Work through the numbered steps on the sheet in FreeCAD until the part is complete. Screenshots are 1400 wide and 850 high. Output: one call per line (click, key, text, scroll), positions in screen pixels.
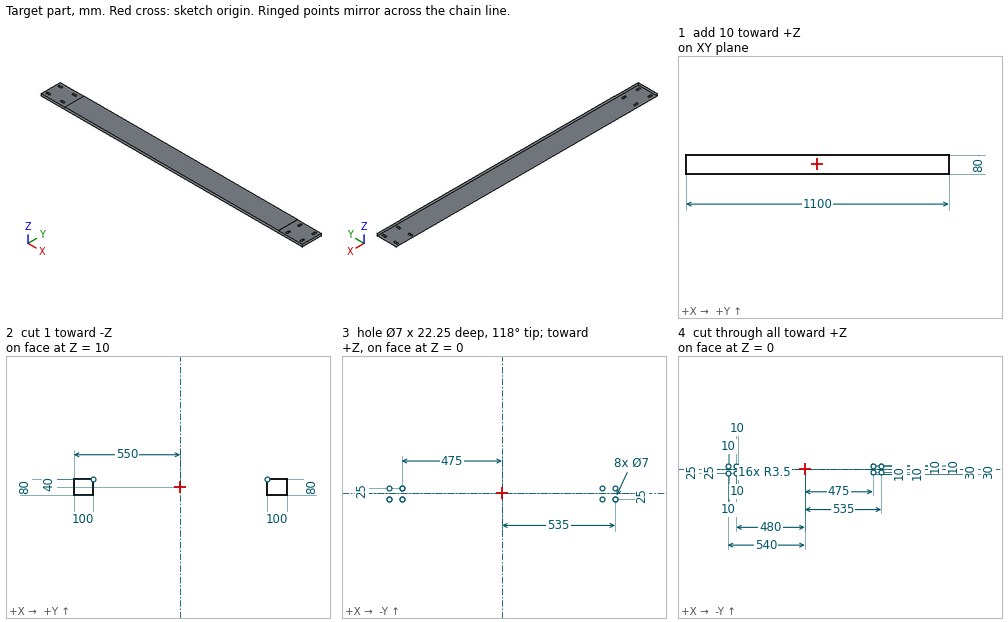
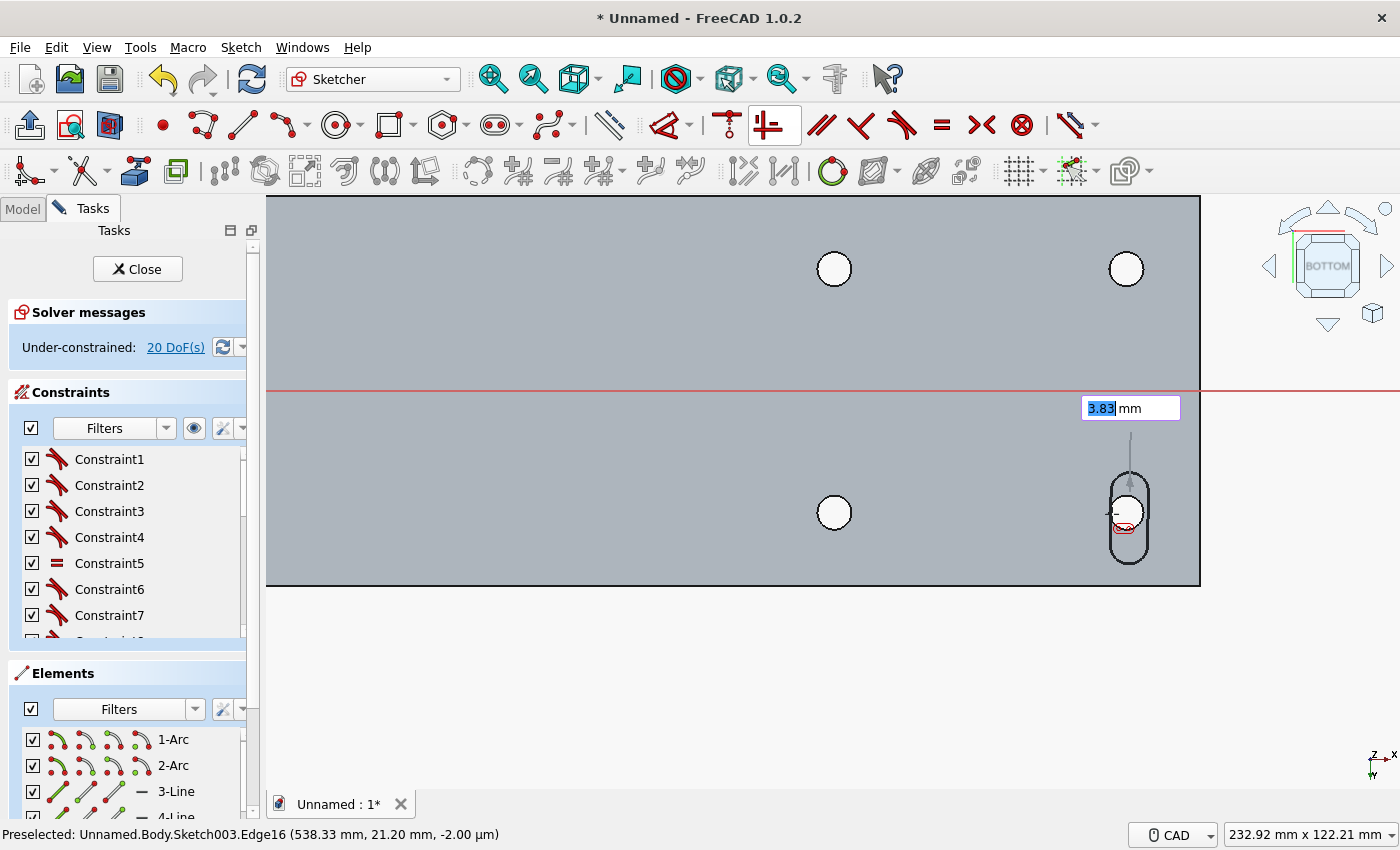
click(1109, 513)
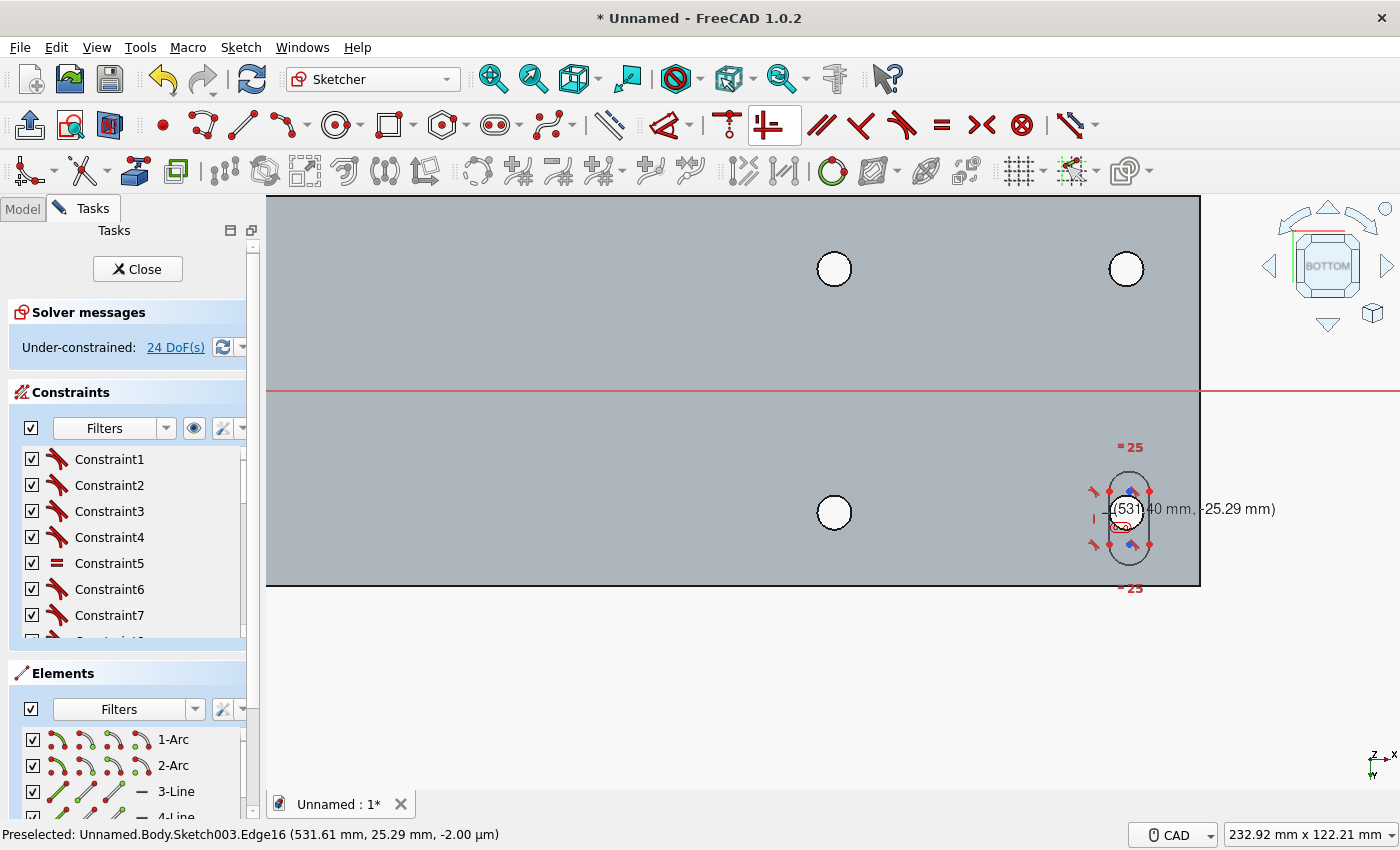
scroll(834, 537, up, 2)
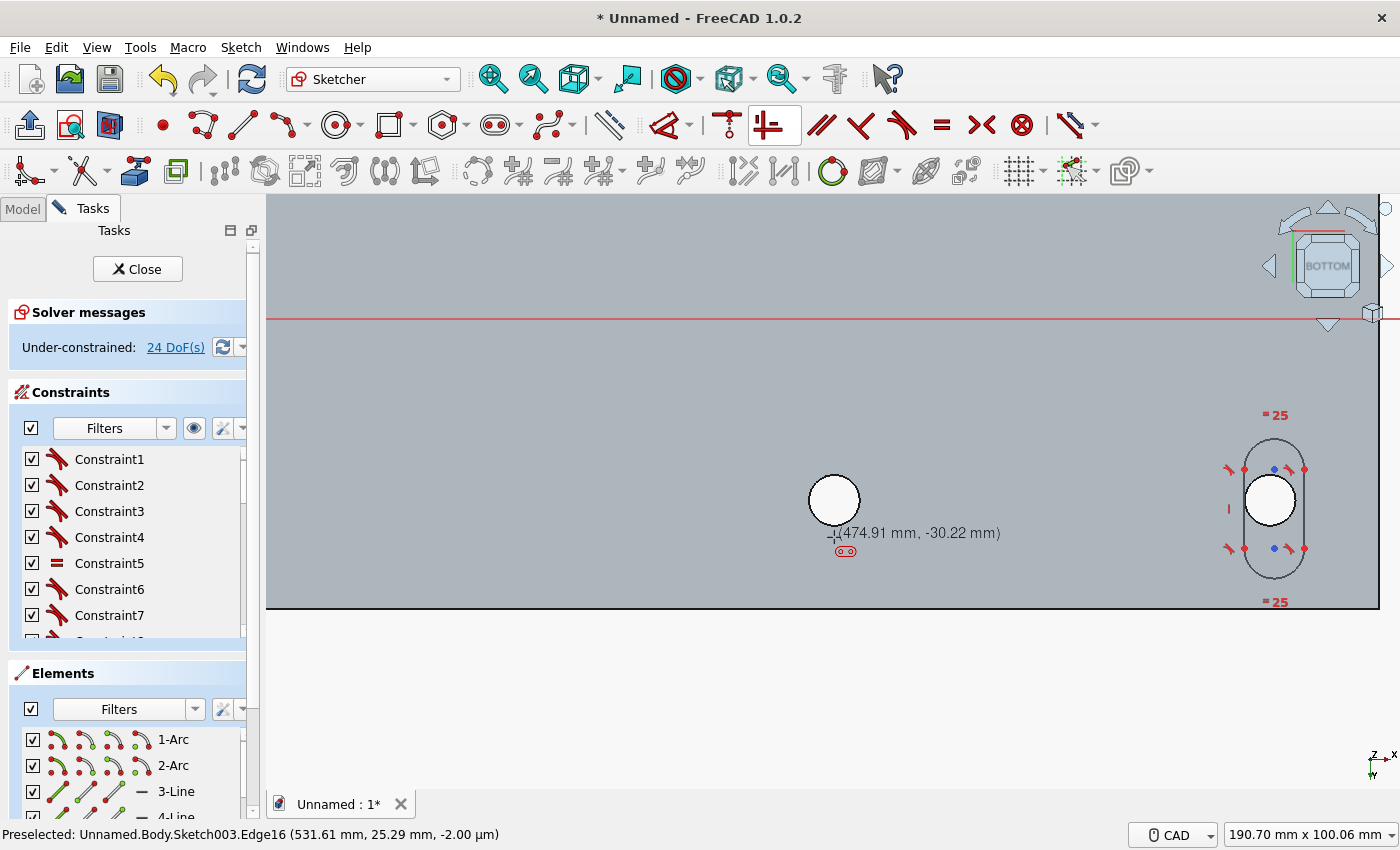
scroll(1104, 509, down, 12)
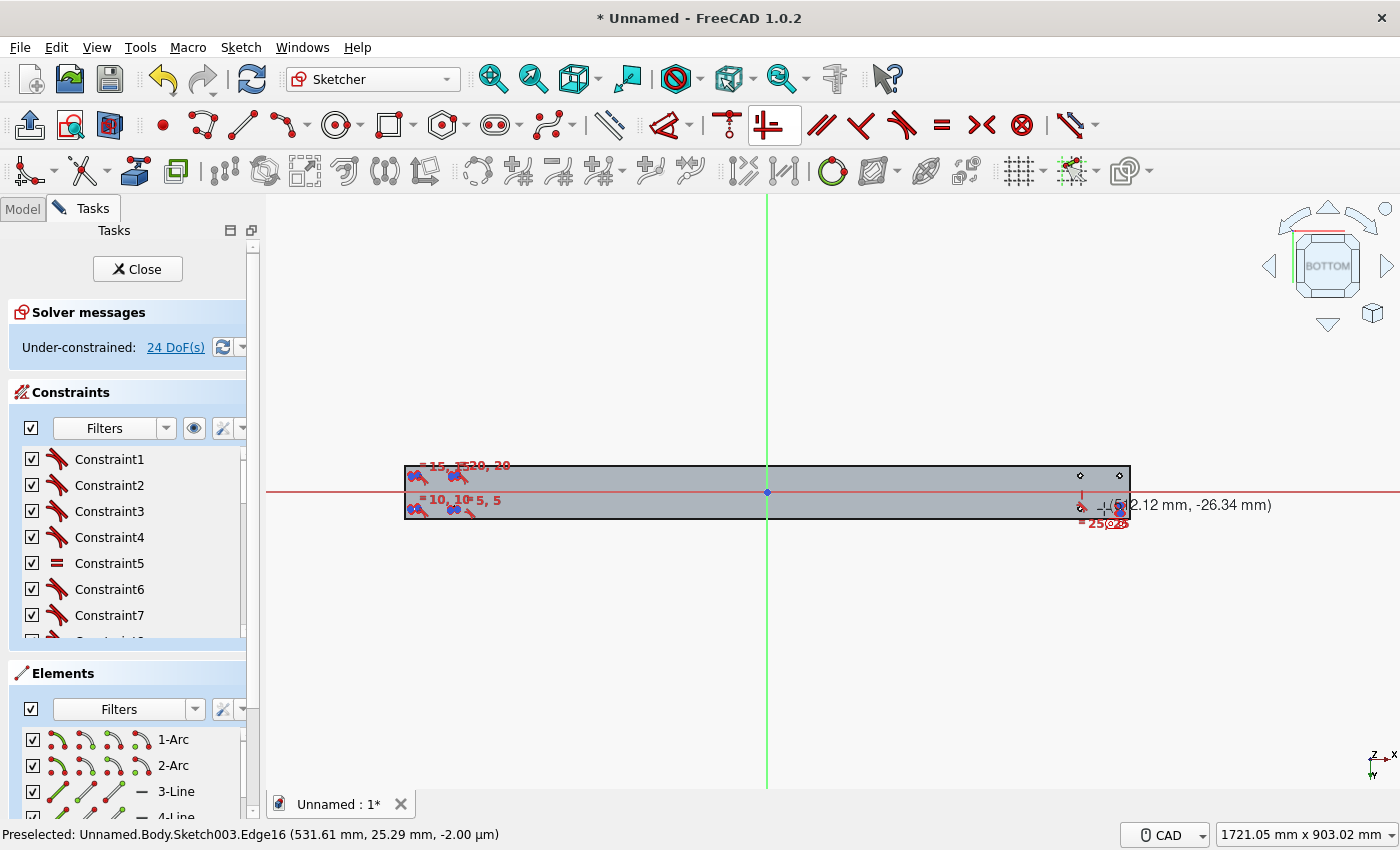
click(1080, 512)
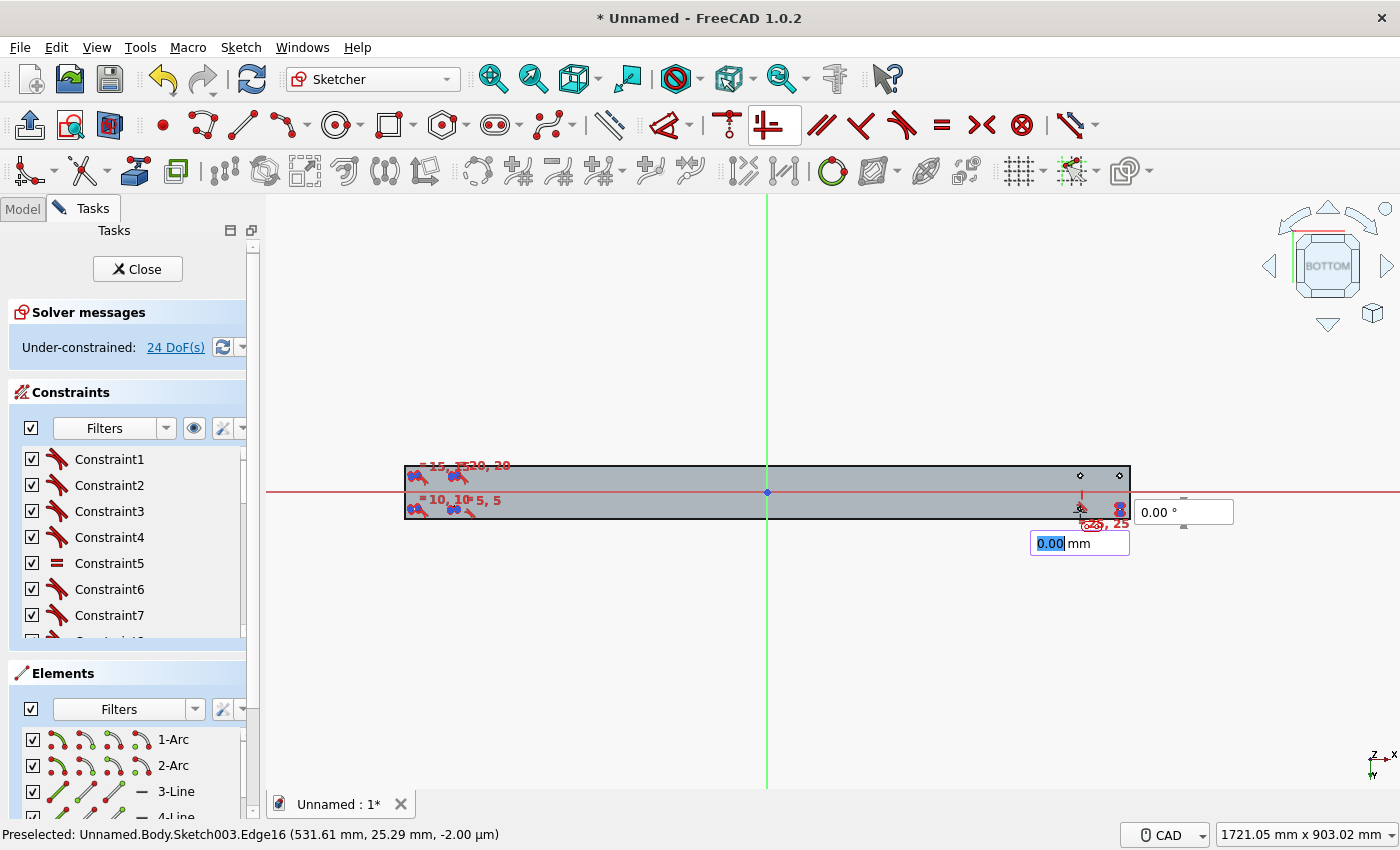
scroll(1080, 505, up, 5)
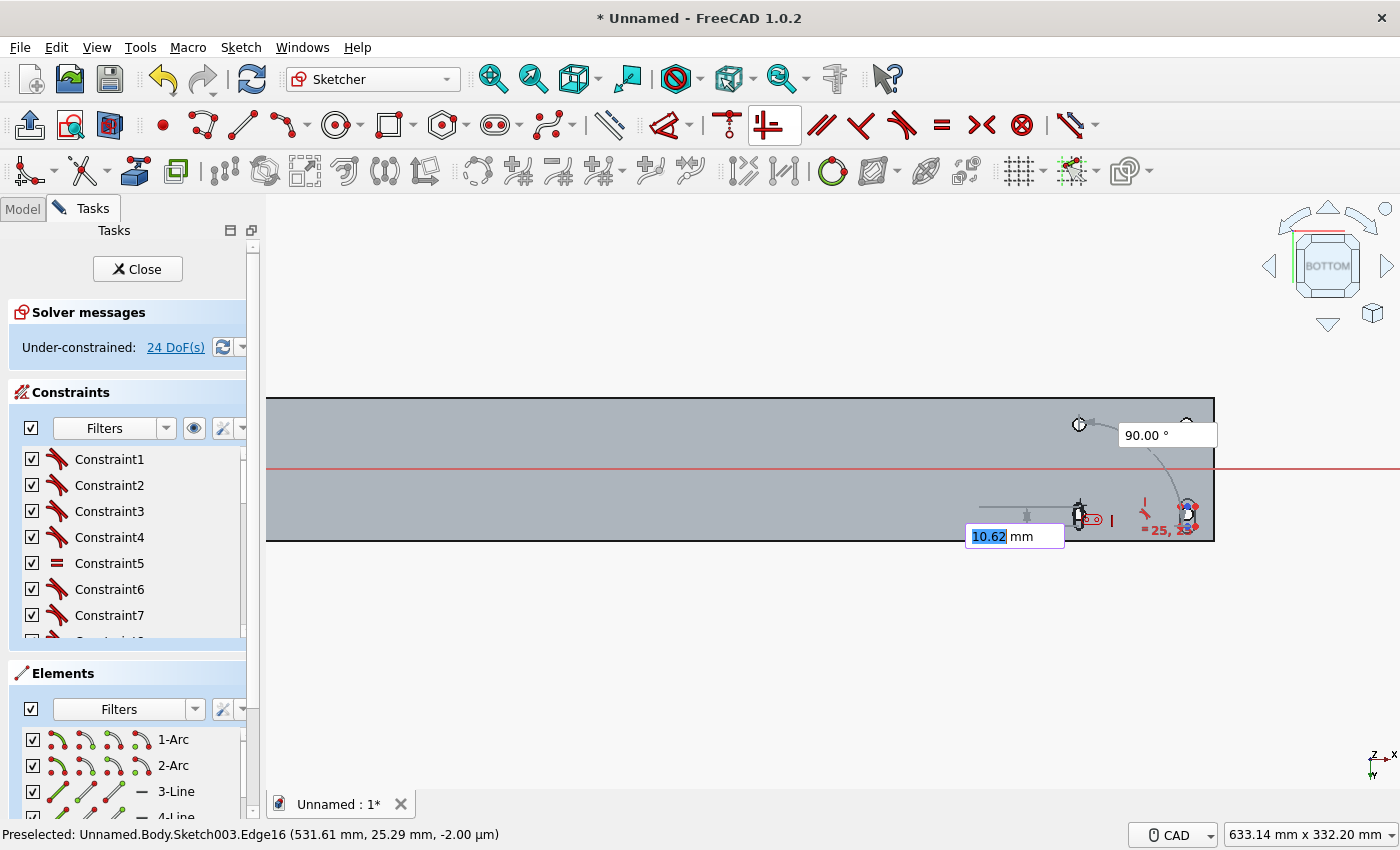
click(1079, 505)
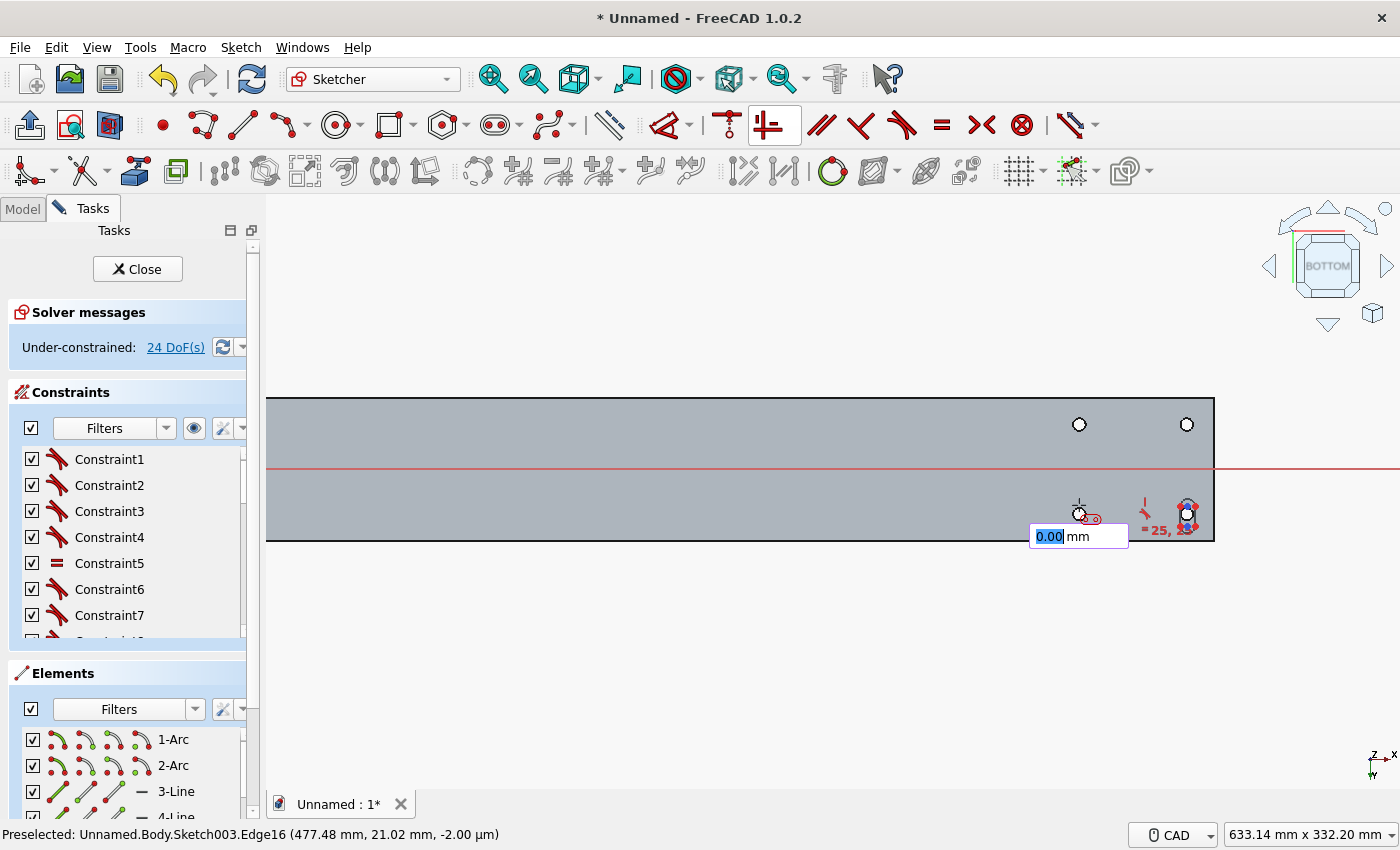
scroll(1073, 514, up, 5)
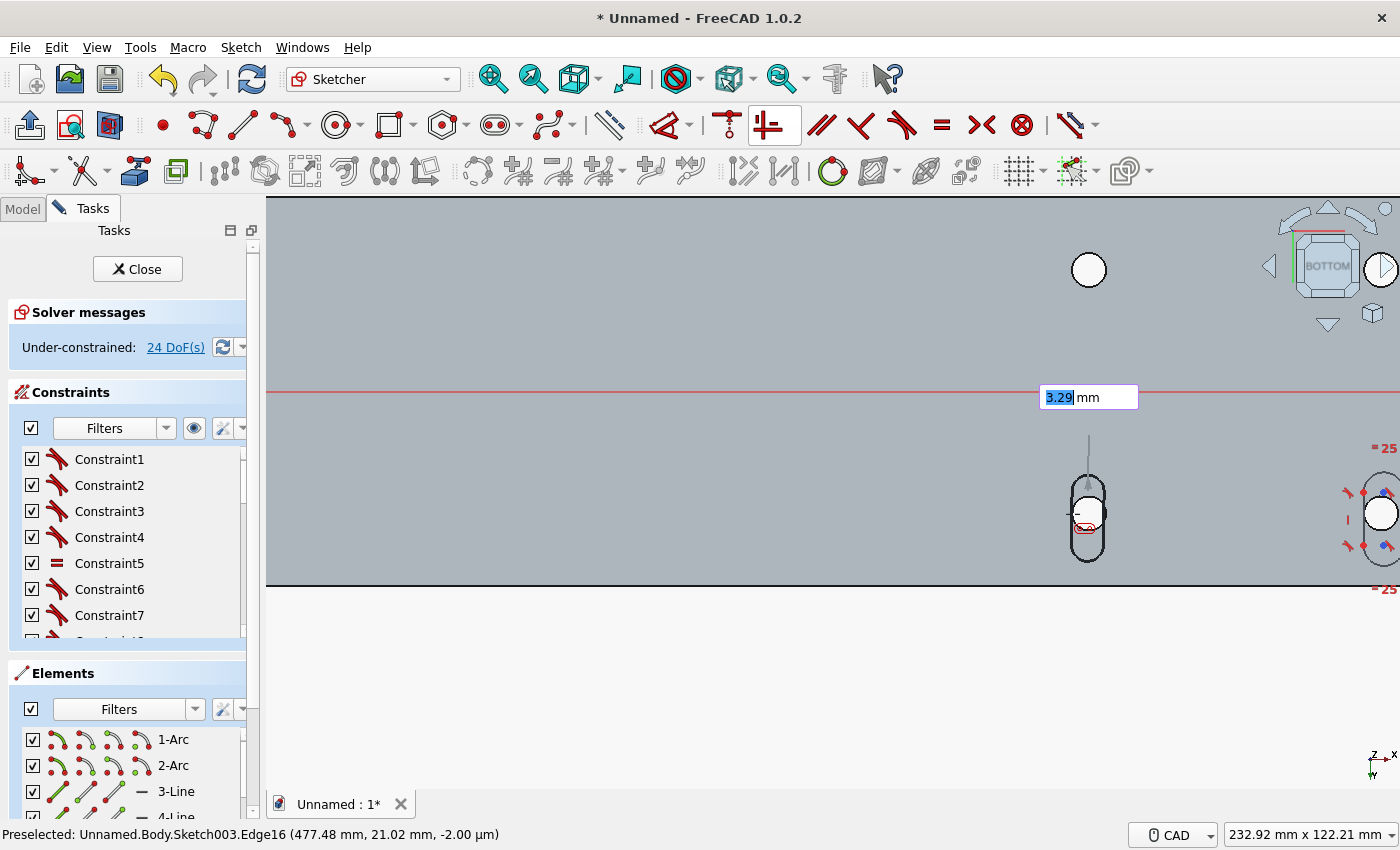
click(1072, 513)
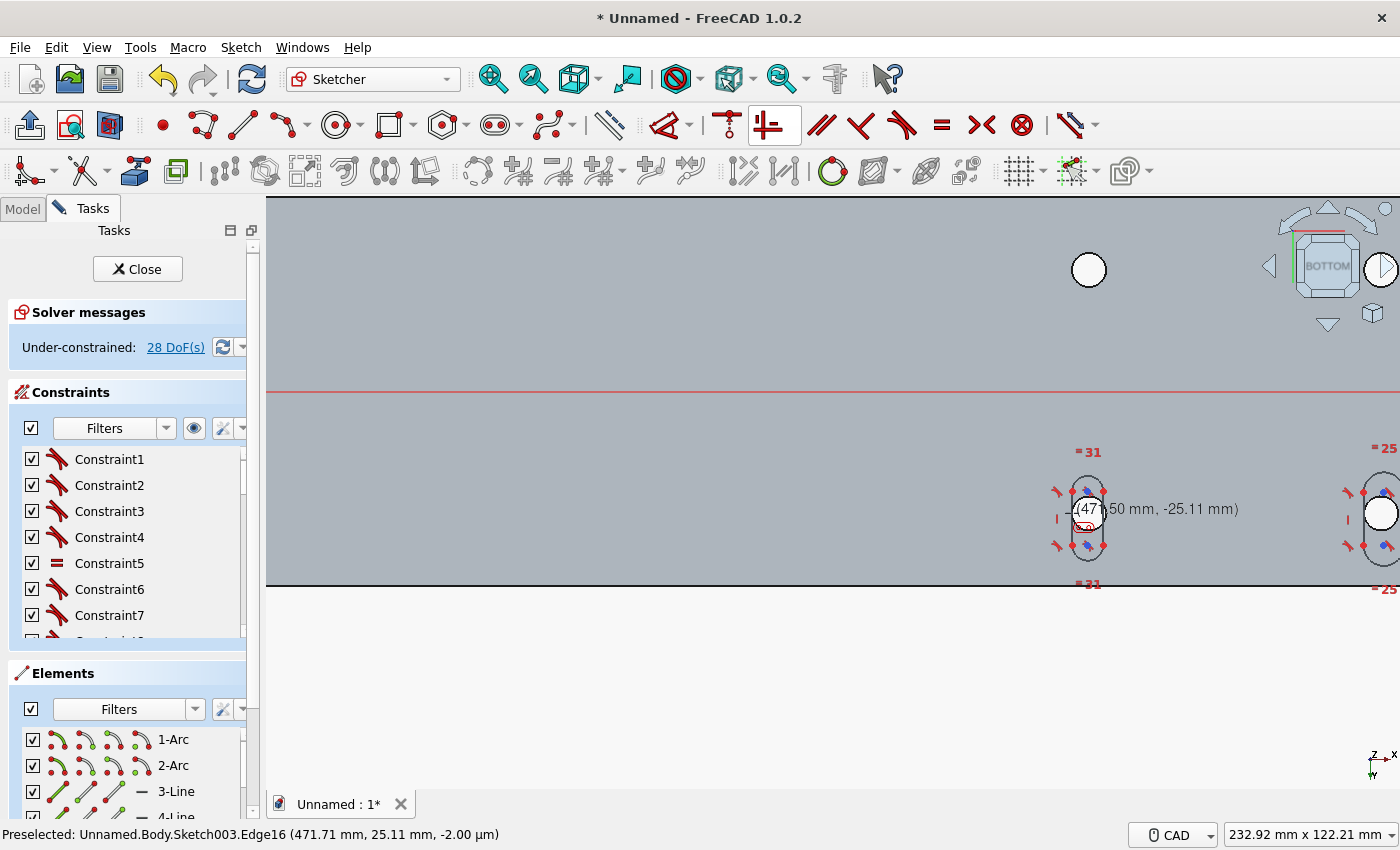
scroll(1078, 507, down, 10)